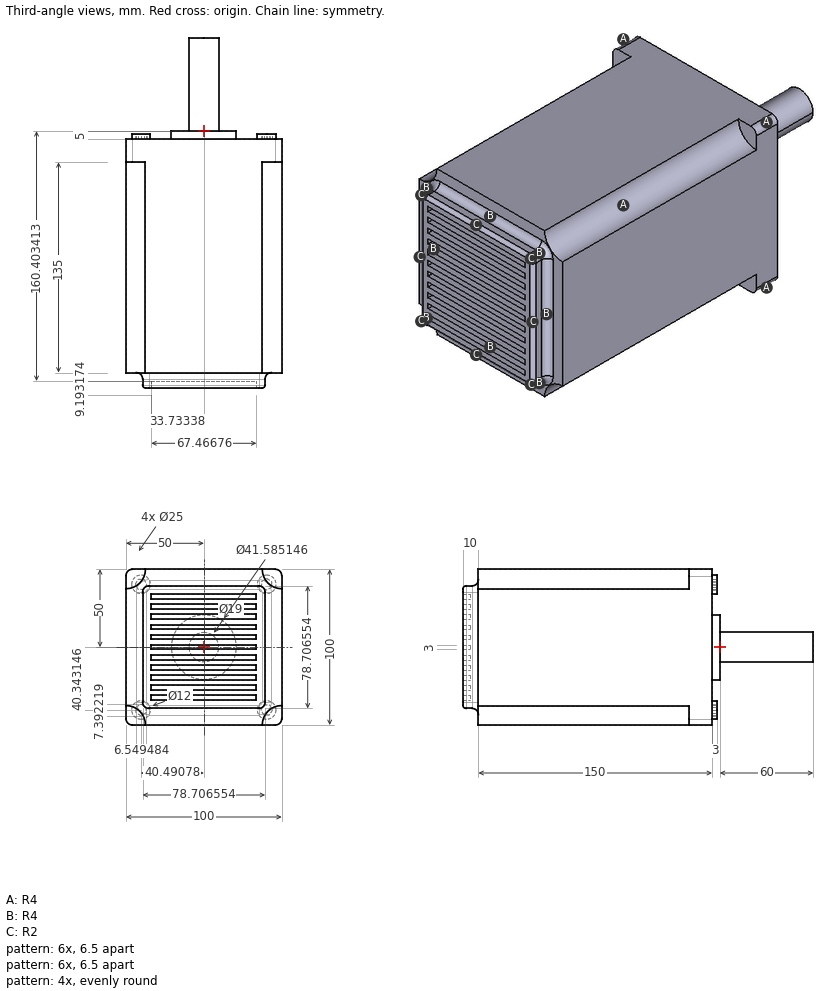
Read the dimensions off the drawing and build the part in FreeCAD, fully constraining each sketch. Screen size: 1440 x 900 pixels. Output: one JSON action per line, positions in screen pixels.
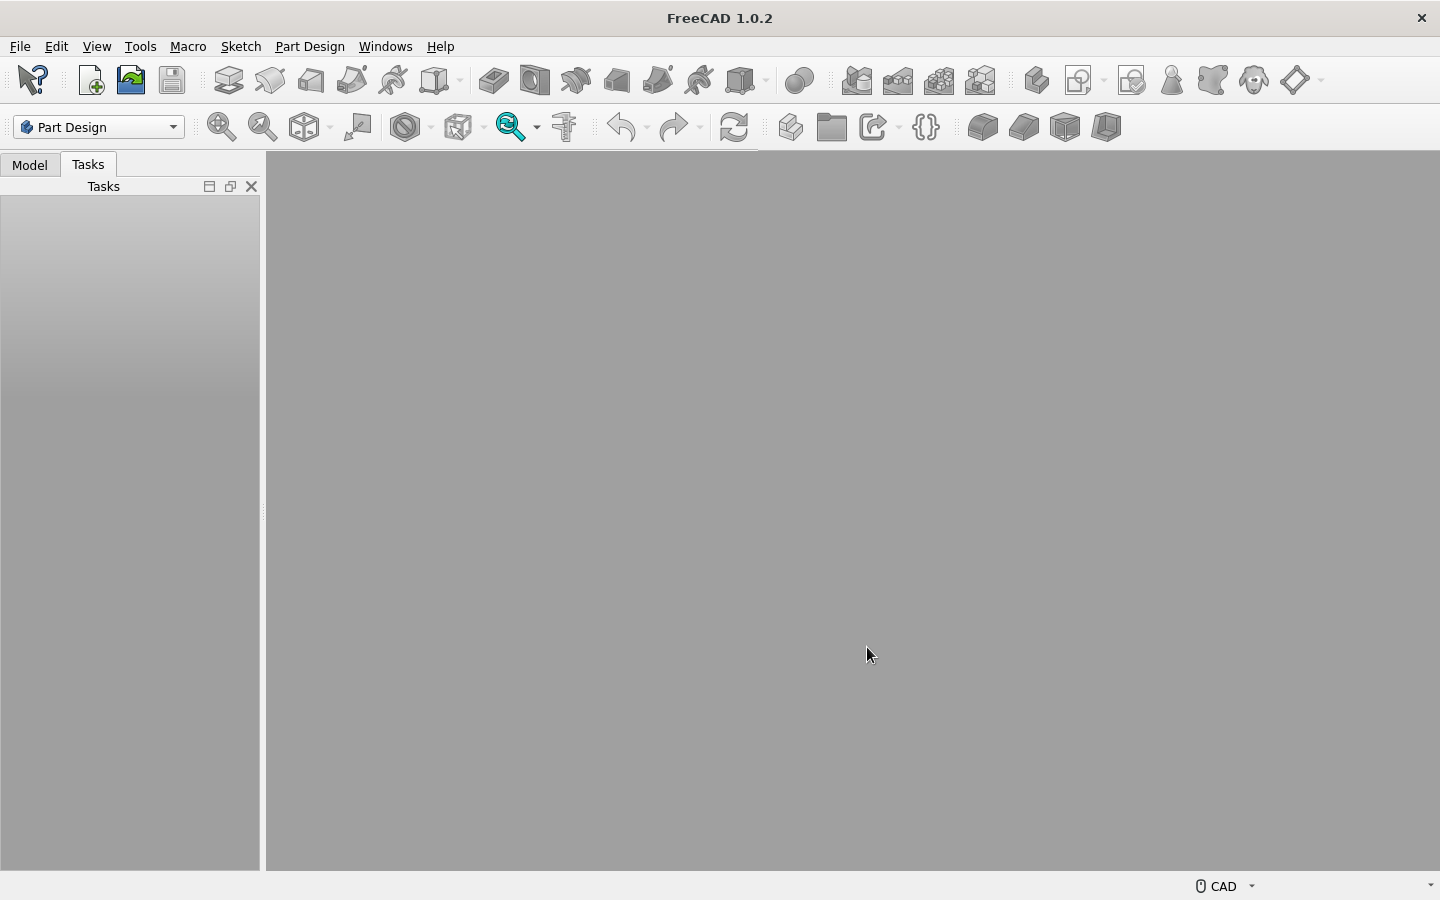
{"action": "key", "text": "ctrl+n"}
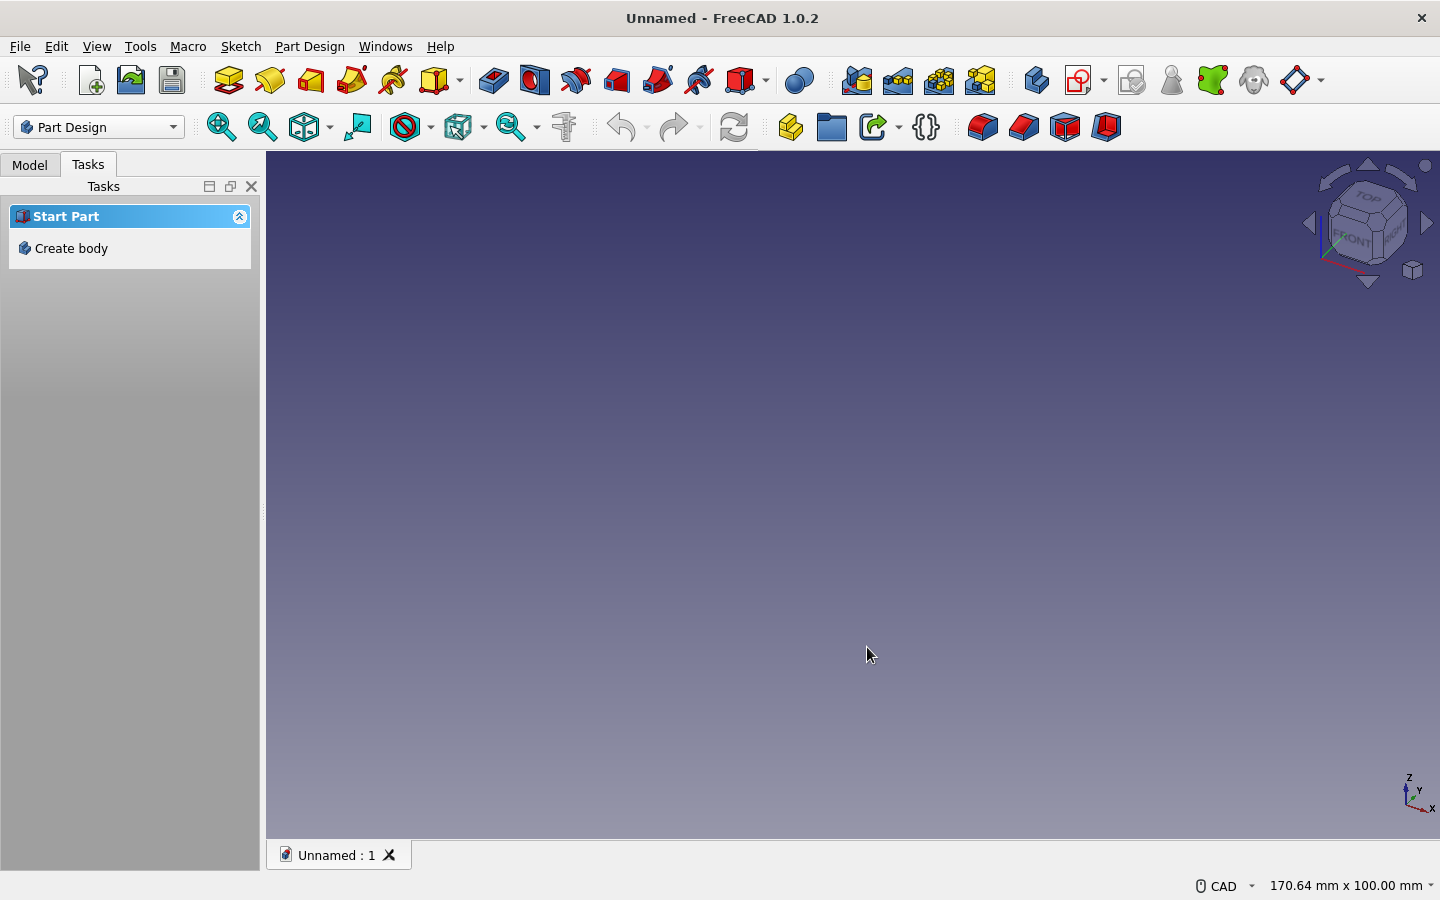
{"action": "left_click", "coordinate": [1078, 80]}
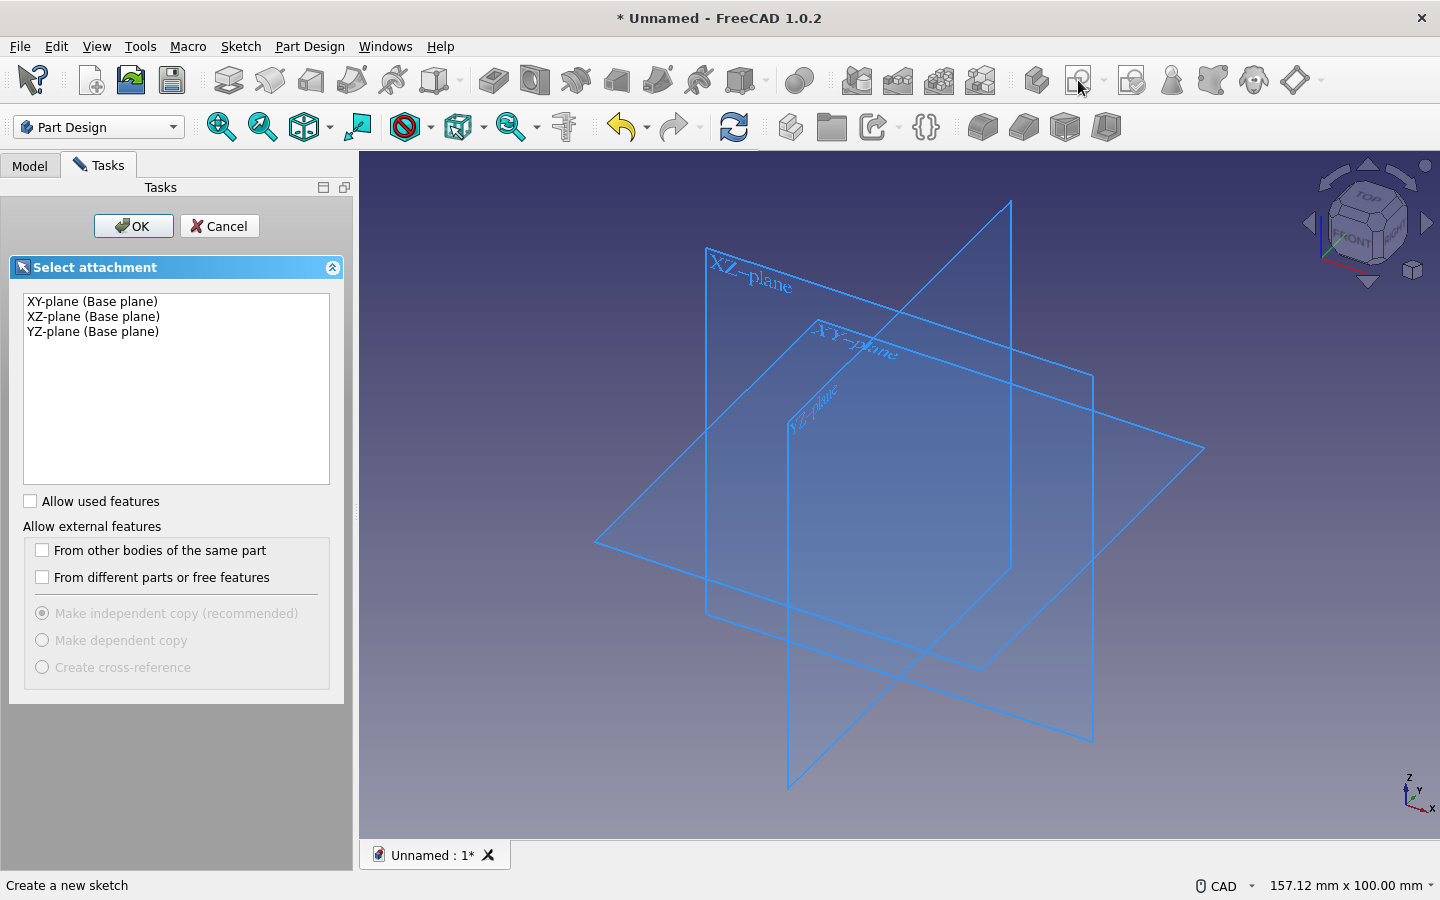
{"action": "left_click", "coordinate": [84, 316]}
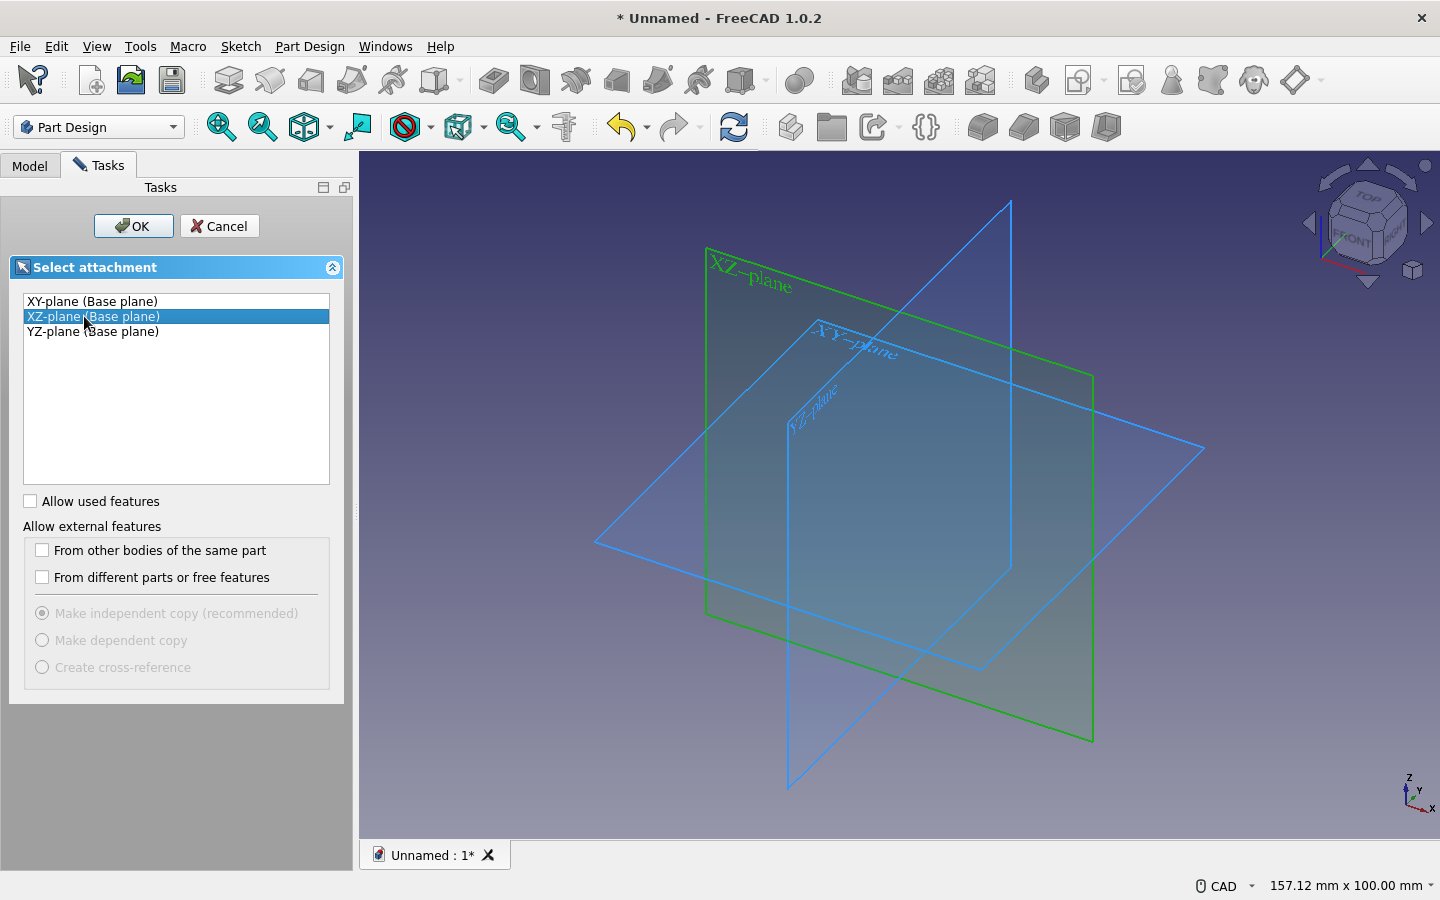
{"action": "left_click", "coordinate": [134, 226]}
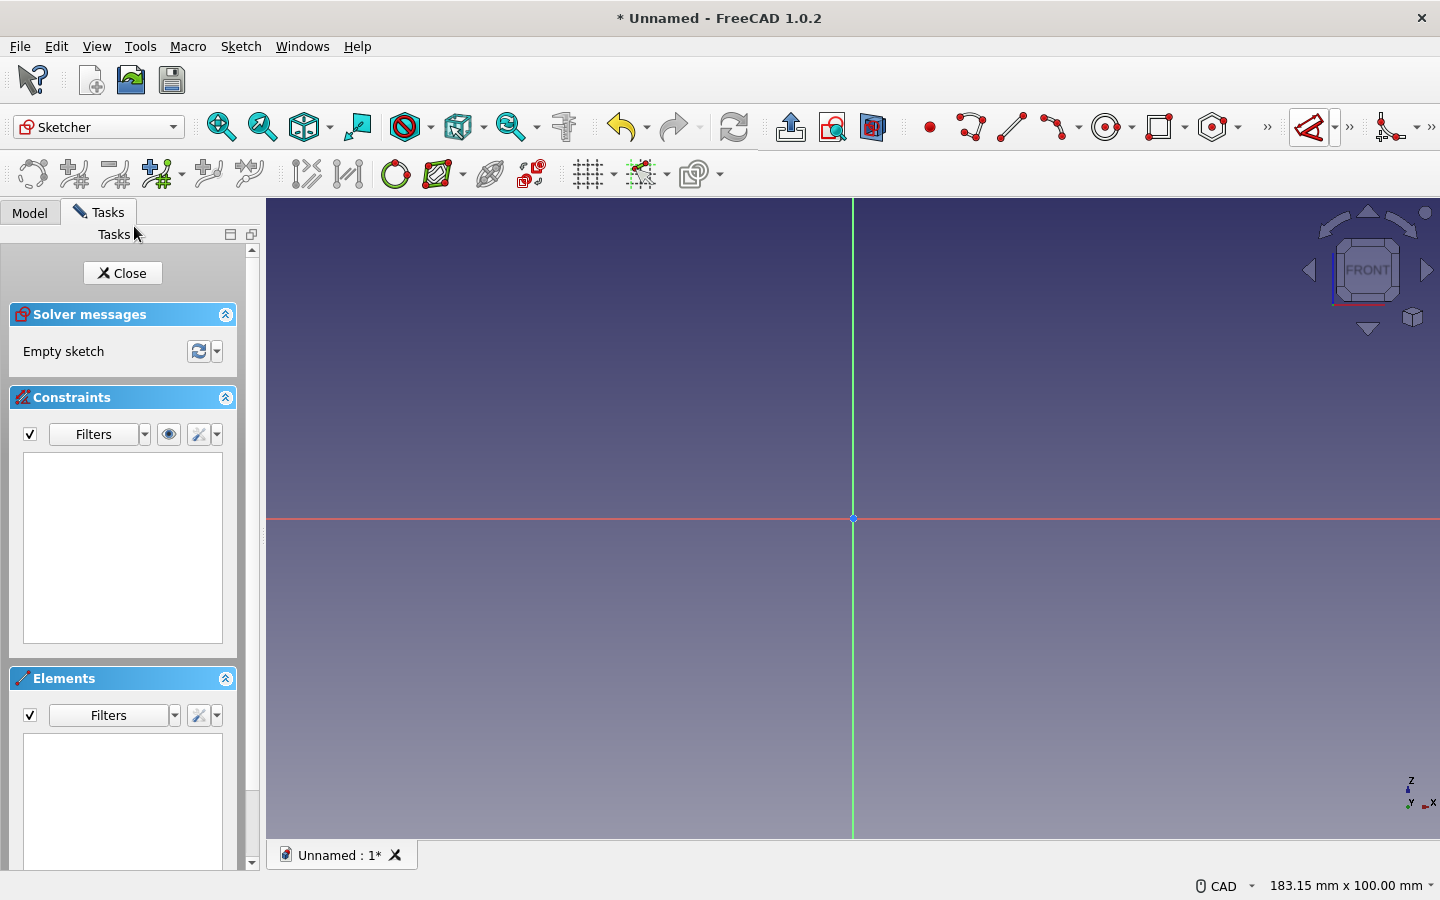
{"action": "scroll", "coordinate": [883, 518], "scroll_direction": "up", "scroll_amount": 6}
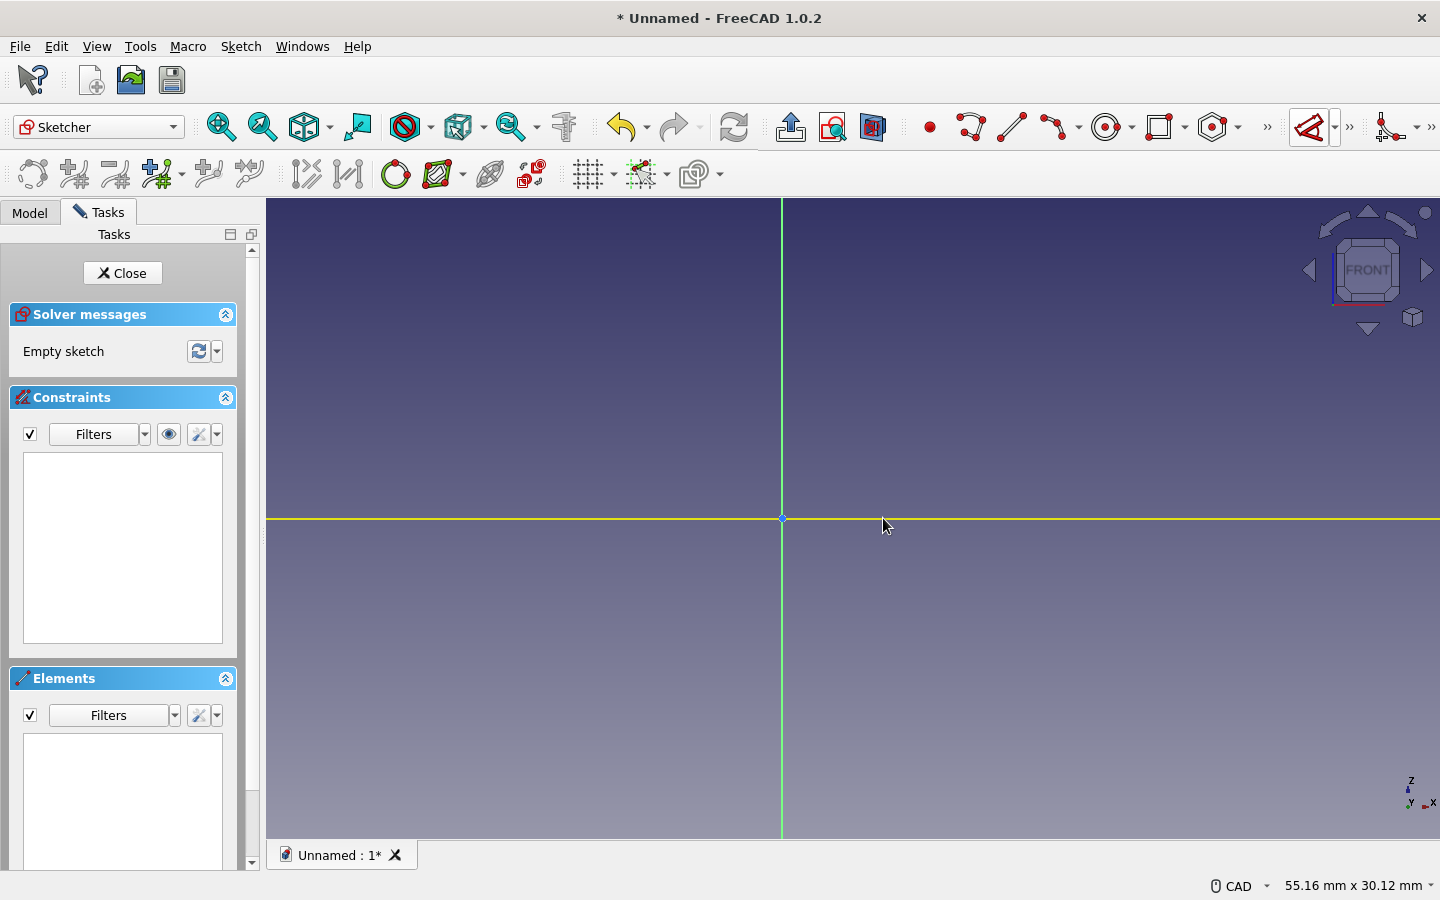
{"action": "left_click", "coordinate": [1106, 128]}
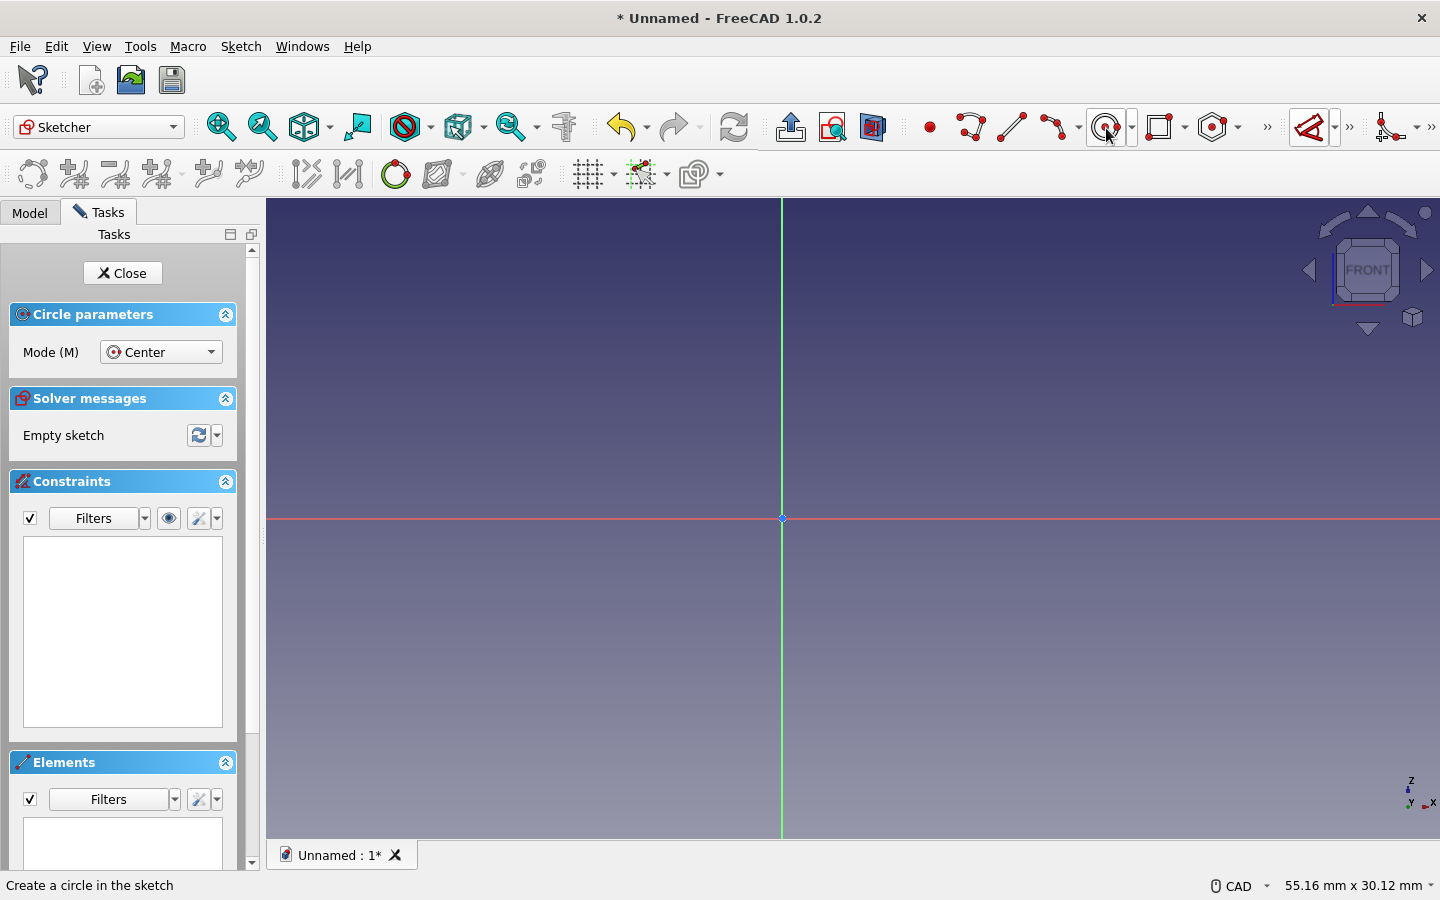
{"action": "left_click", "coordinate": [782, 518]}
{"action": "left_click", "coordinate": [925, 376]}
{"action": "key", "text": "Escape"}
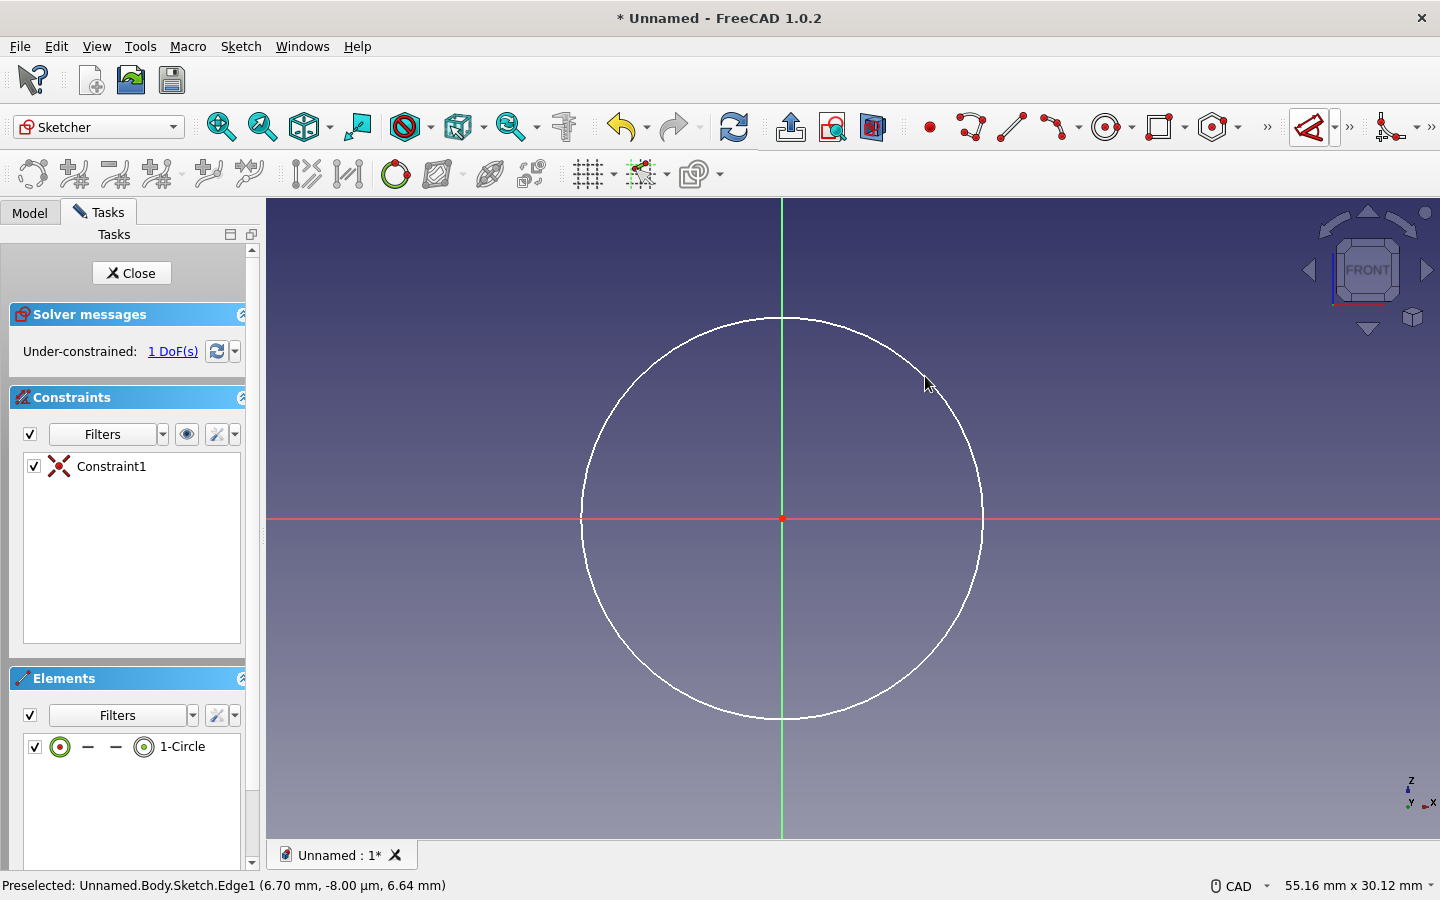
{"action": "left_click", "coordinate": [1308, 128]}